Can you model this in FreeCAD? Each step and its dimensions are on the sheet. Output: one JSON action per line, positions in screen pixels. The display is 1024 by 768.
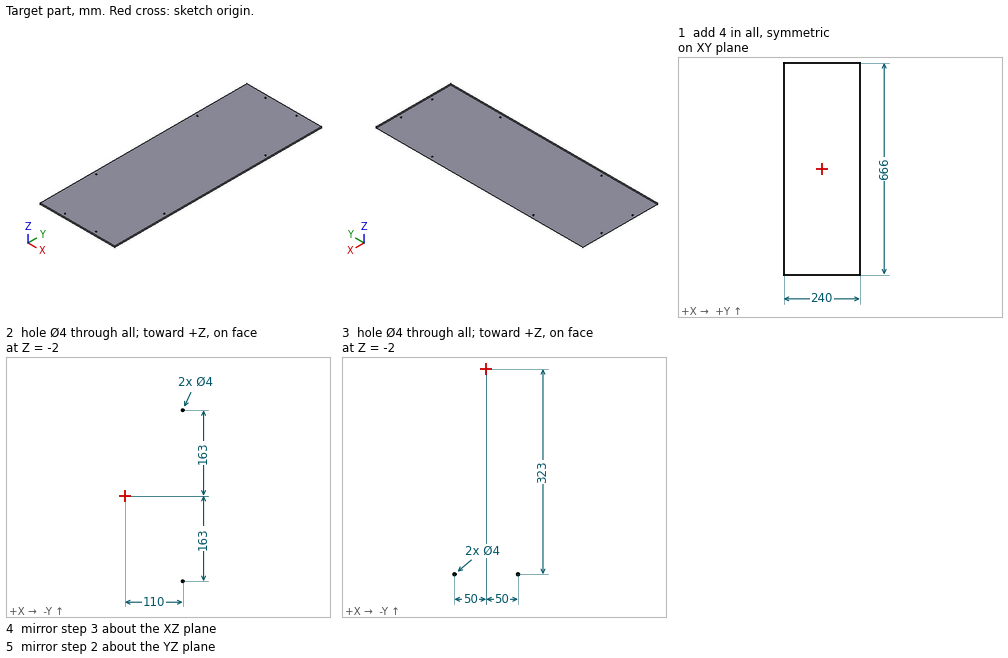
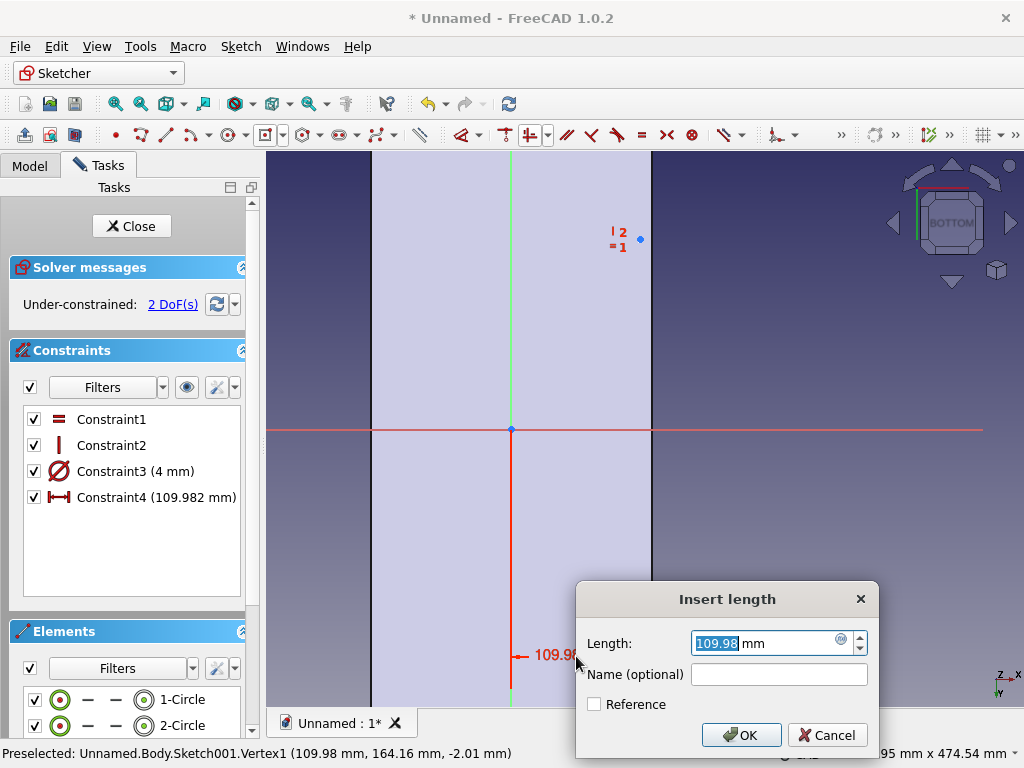
{"action": "type", "text": "110"}
{"action": "key", "text": "Return"}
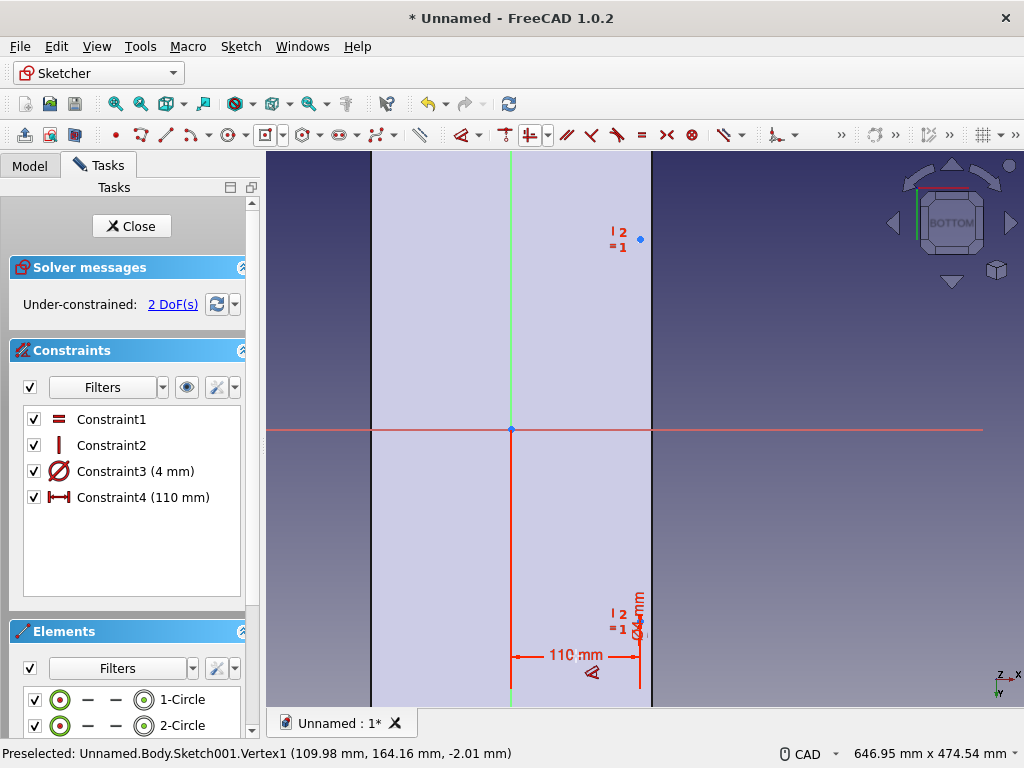
{"action": "left_click", "coordinate": [640, 622]}
{"action": "left_click", "coordinate": [477, 526]}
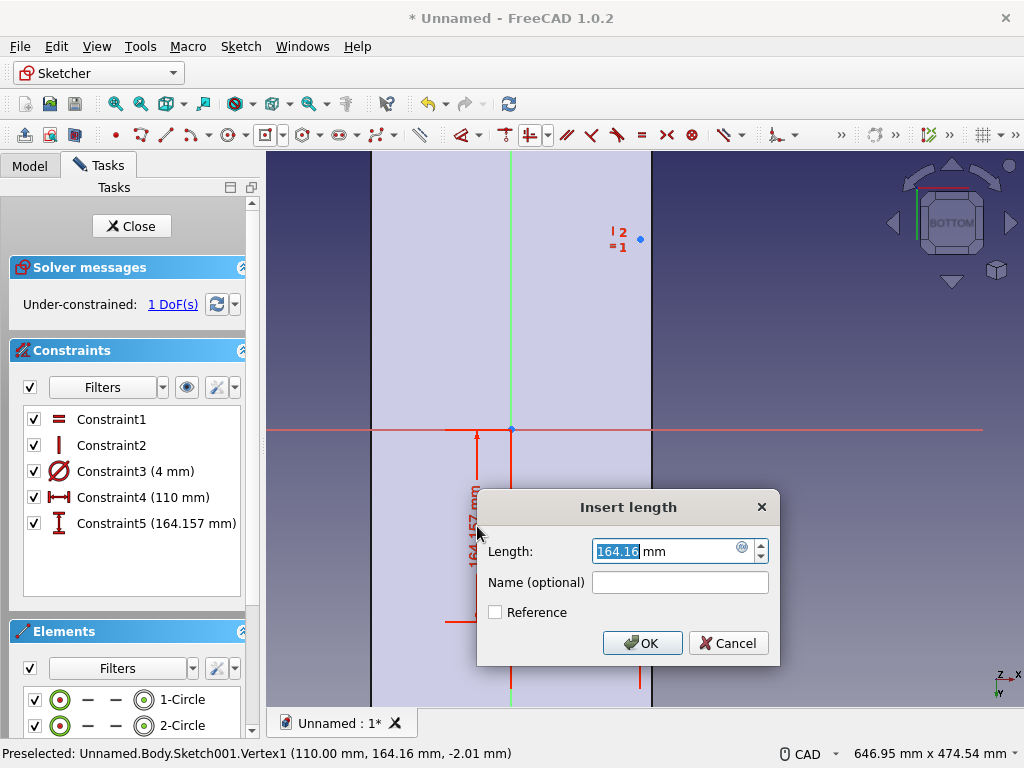
{"action": "type", "text": "163"}
{"action": "key", "text": "Return"}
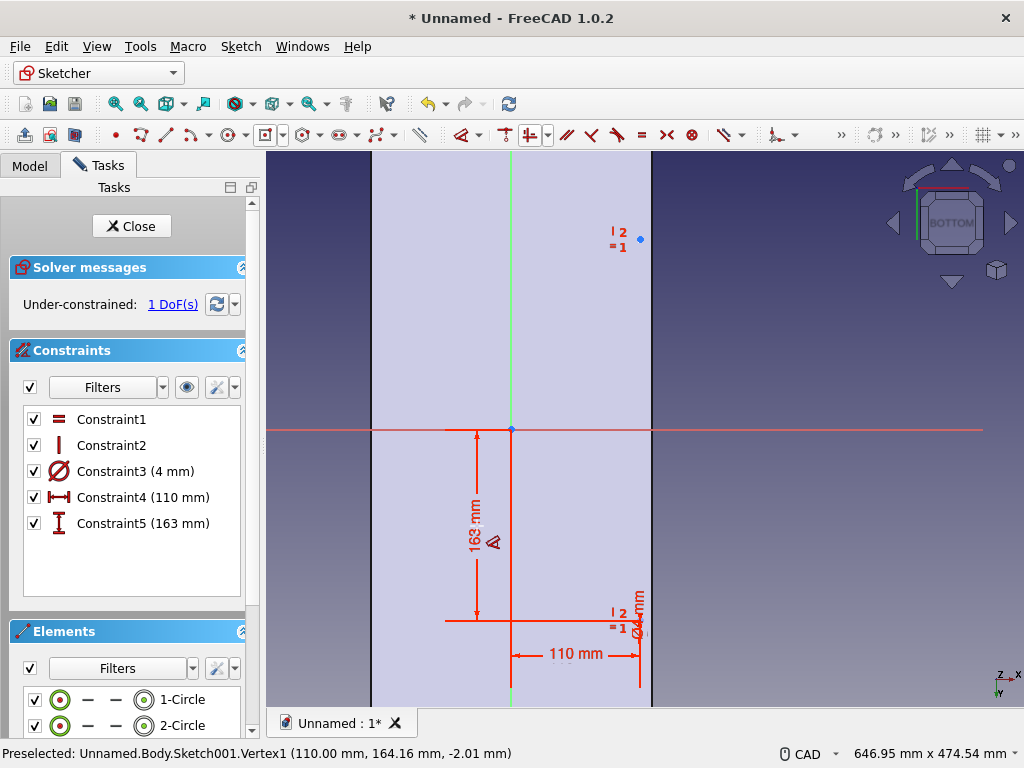
{"action": "left_click", "coordinate": [640, 240]}
{"action": "left_click", "coordinate": [477, 335]}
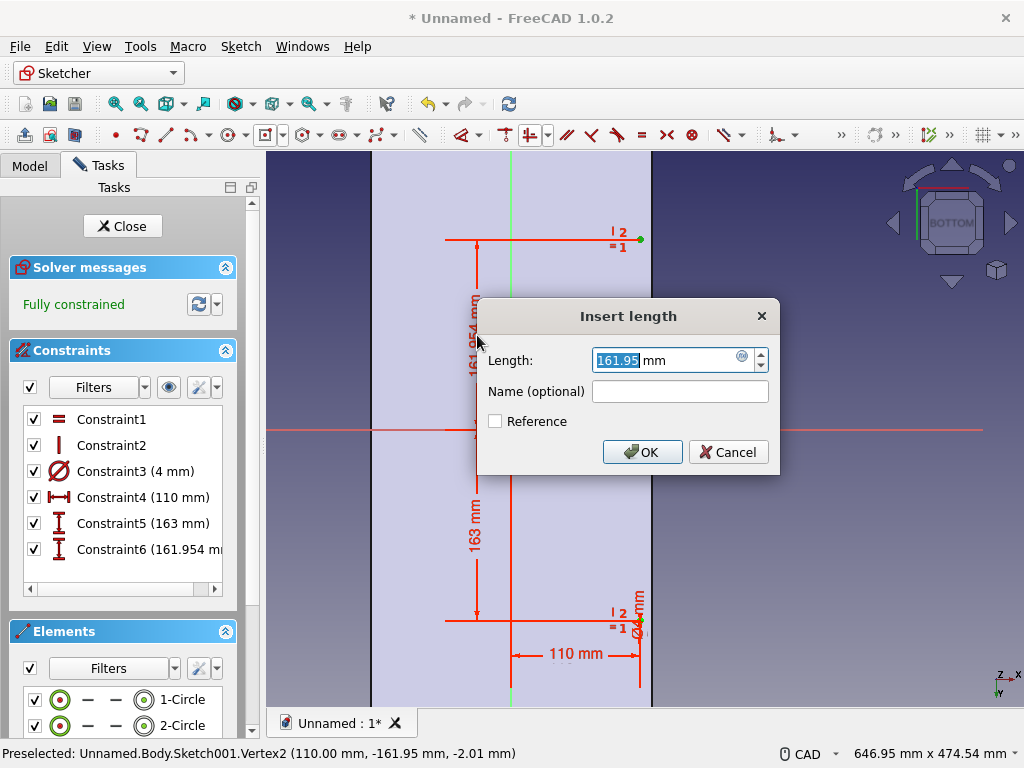
{"action": "type", "text": "163"}
{"action": "key", "text": "Return"}
{"action": "key", "text": "Escape"}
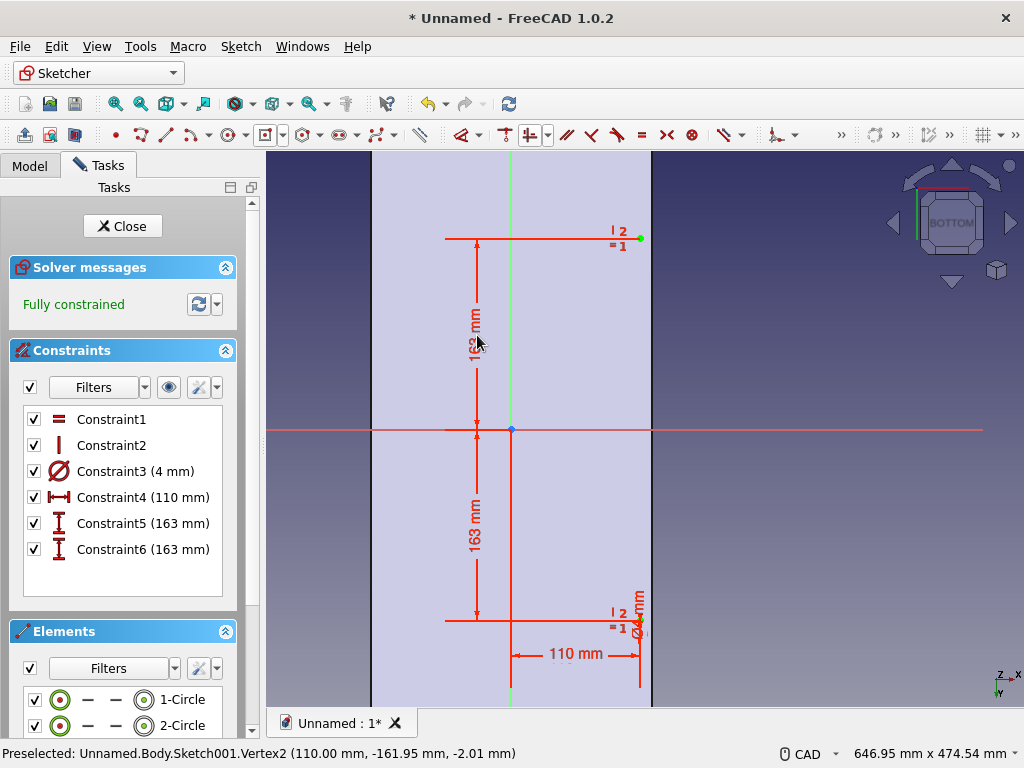
{"action": "left_click", "coordinate": [123, 226]}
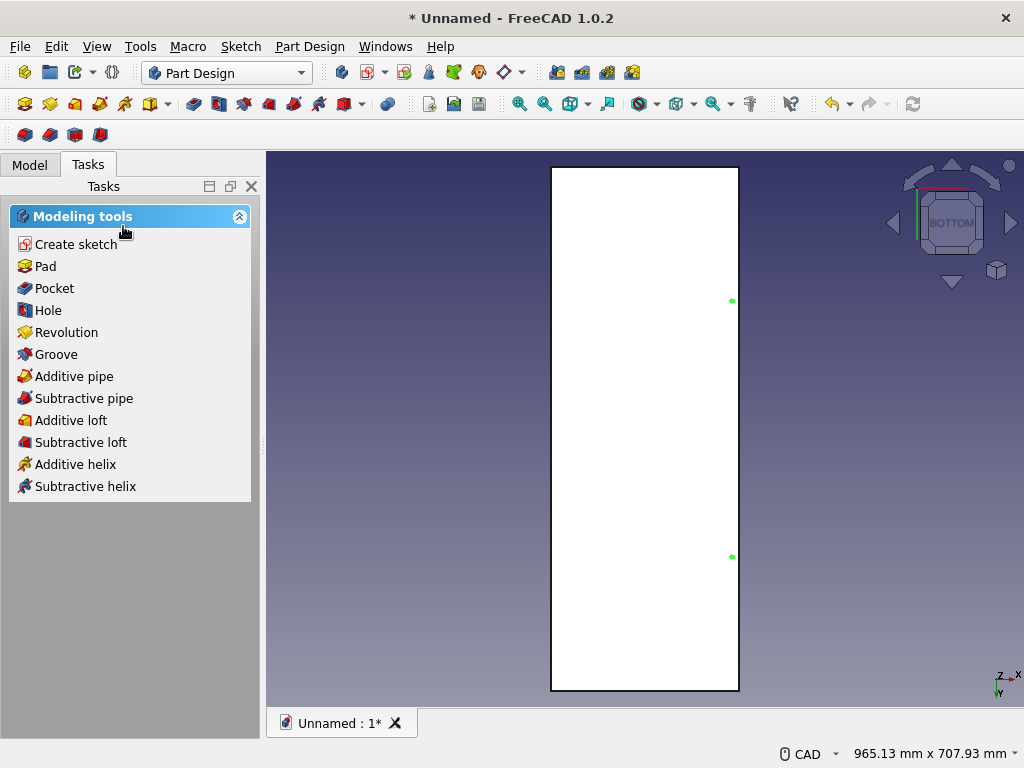
{"action": "left_click", "coordinate": [219, 104]}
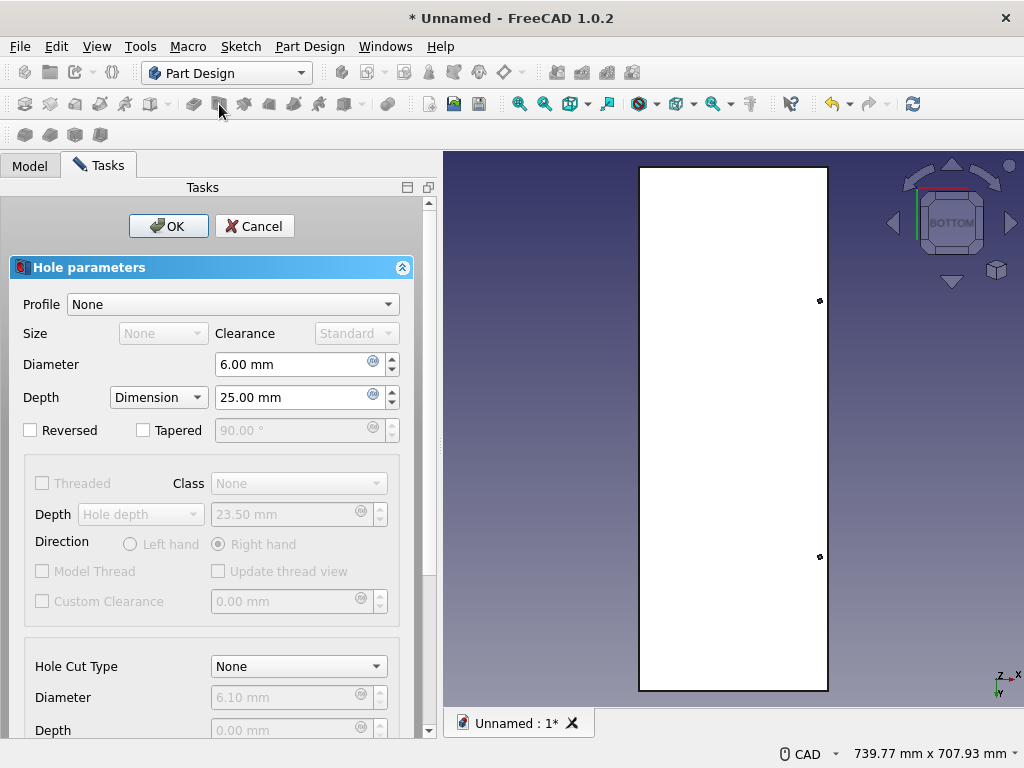
{"action": "triple_click", "coordinate": [300, 364]}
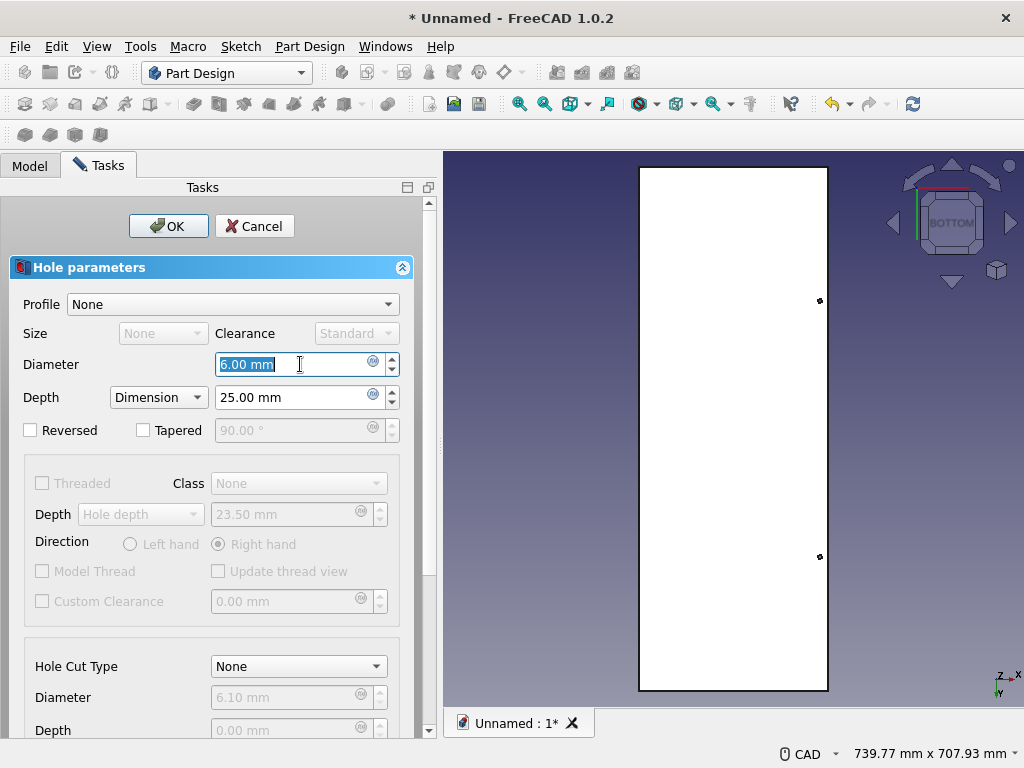
{"action": "type", "text": "4"}
{"action": "key", "text": "Tab"}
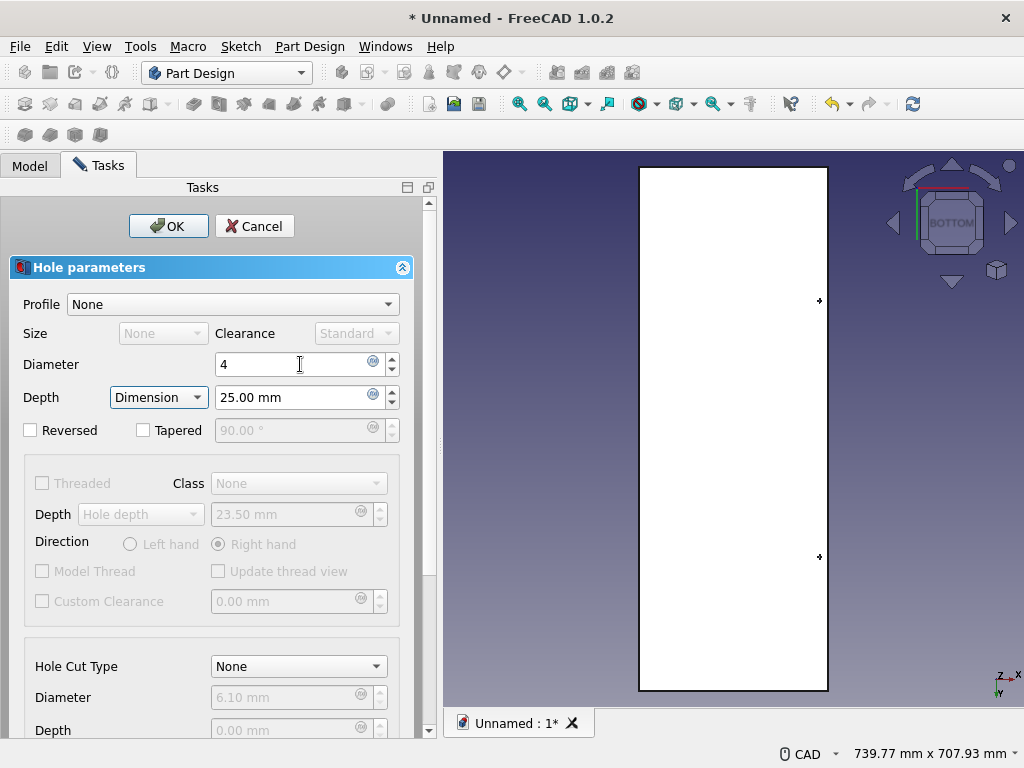
{"action": "left_click", "coordinate": [160, 398]}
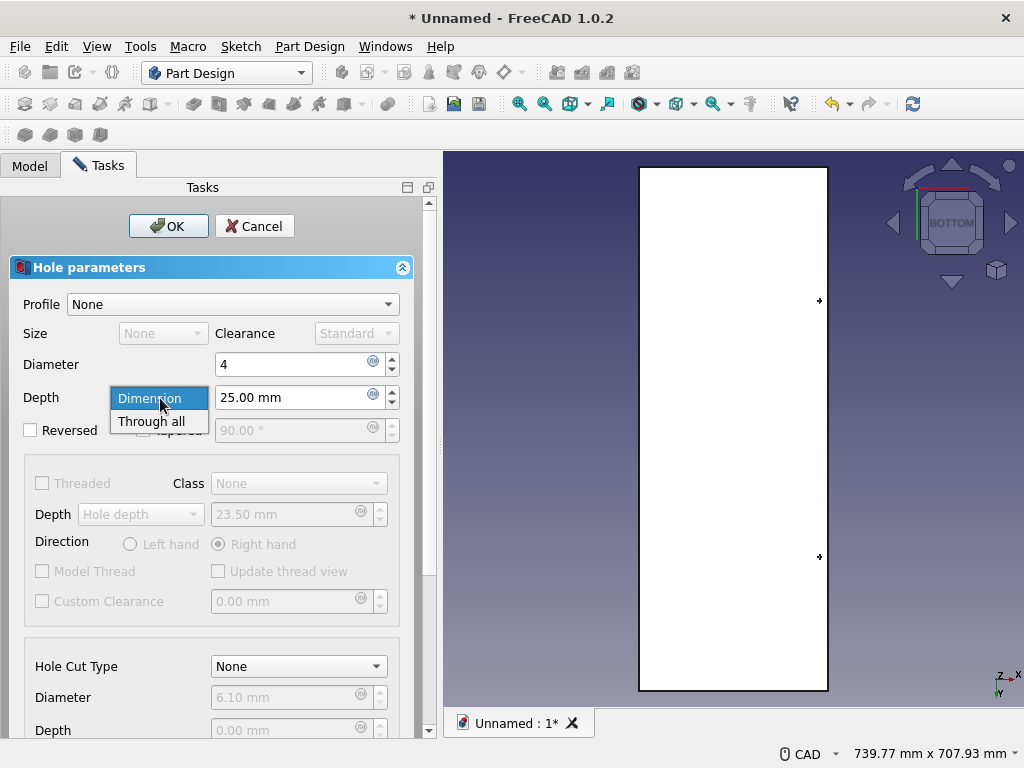
{"action": "left_click", "coordinate": [158, 422]}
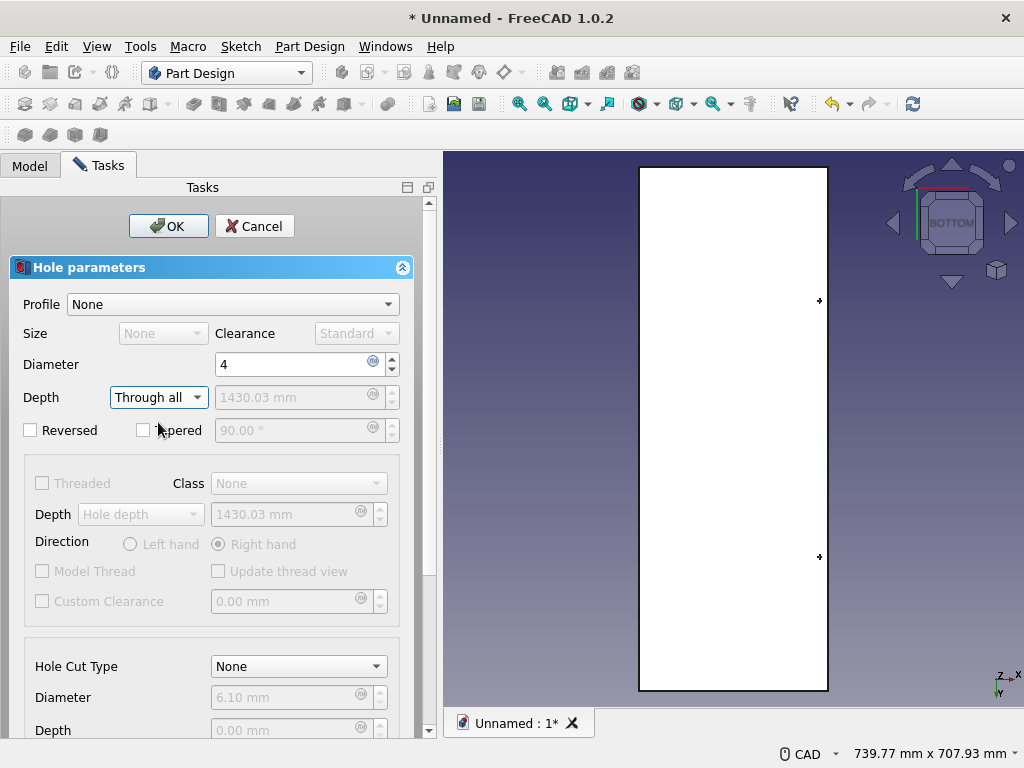
{"action": "left_click", "coordinate": [169, 226]}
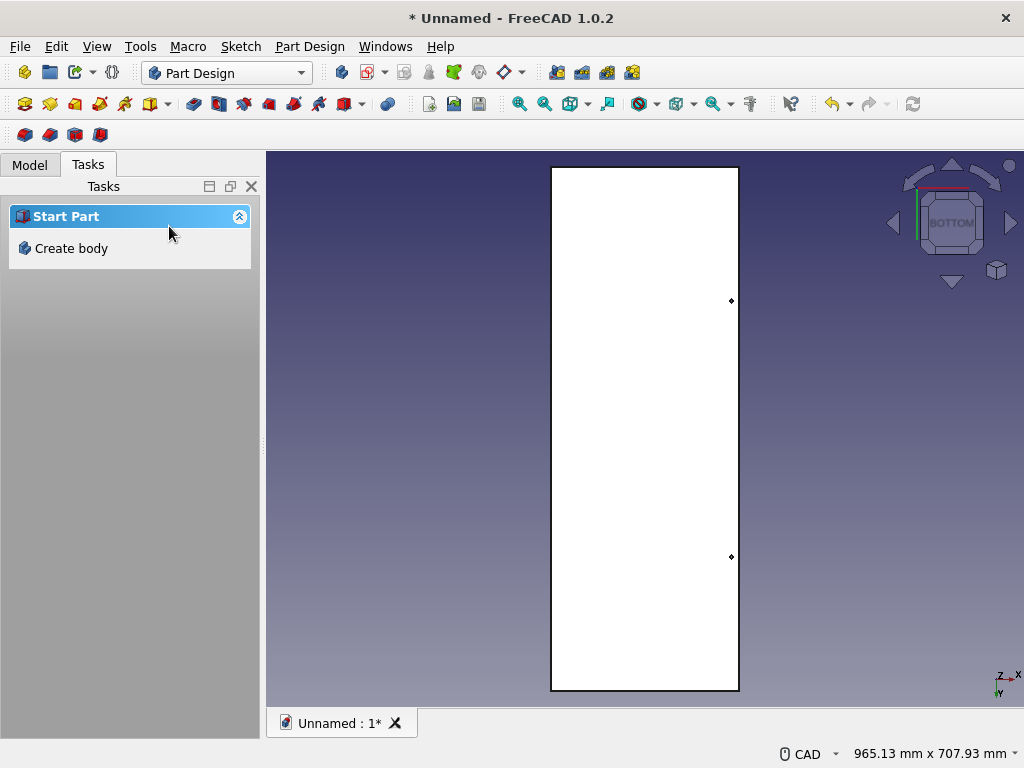
{"action": "left_click", "coordinate": [645, 503]}